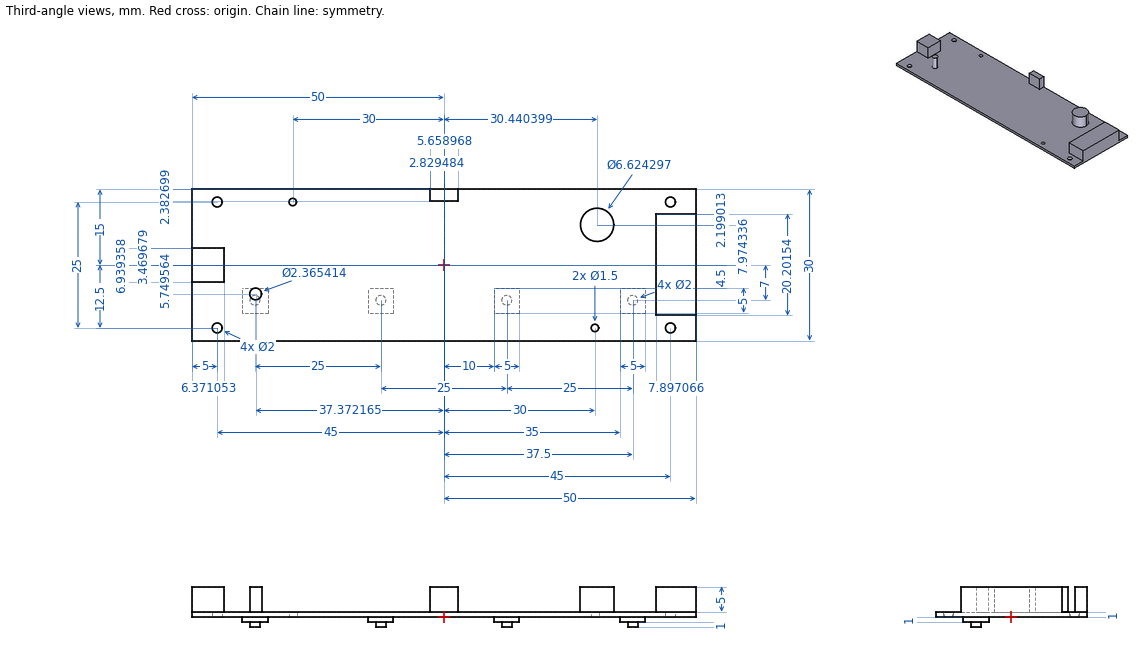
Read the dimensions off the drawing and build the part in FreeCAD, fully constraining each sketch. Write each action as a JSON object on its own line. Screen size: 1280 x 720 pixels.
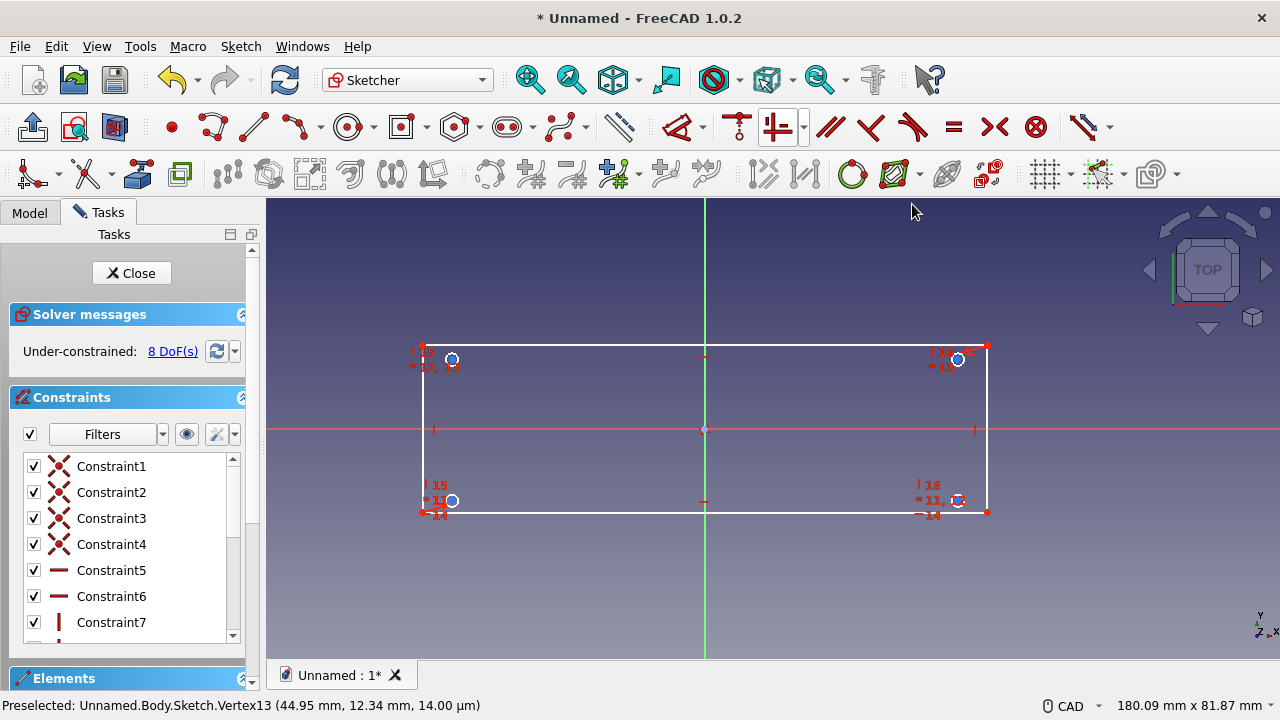
{"action": "scroll", "coordinate": [452, 360], "scroll_direction": "up", "scroll_amount": 4}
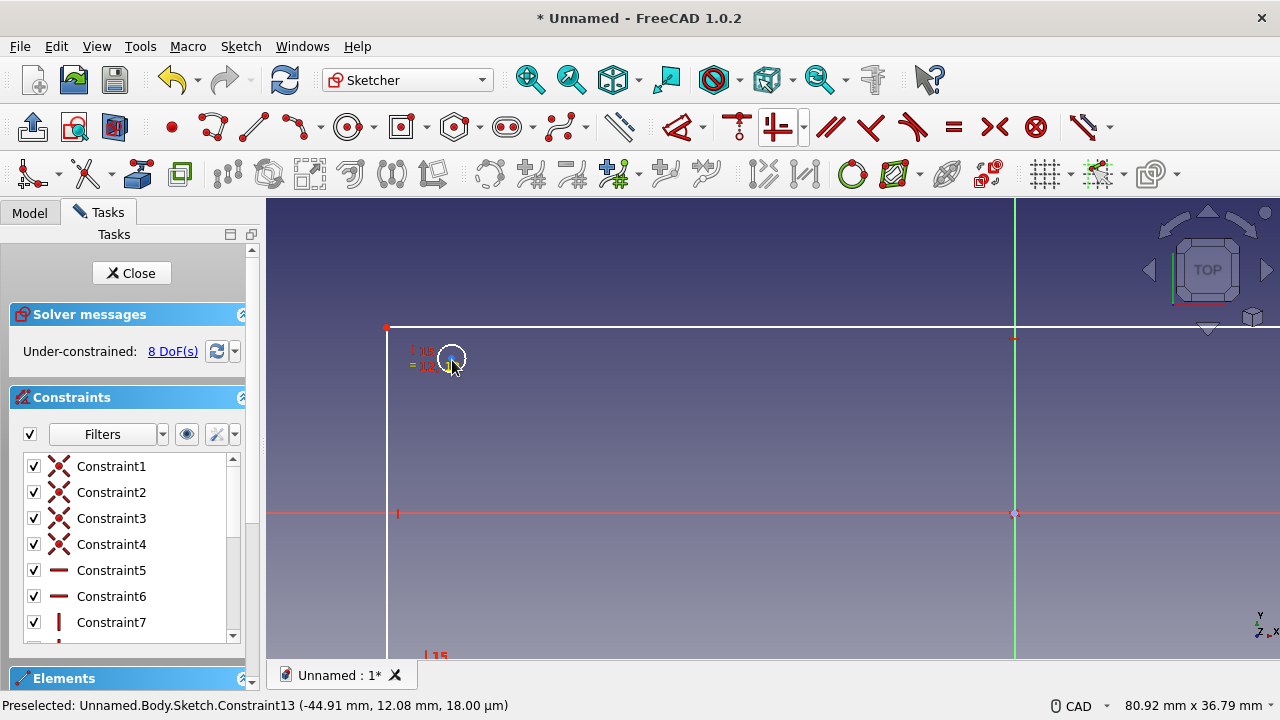
{"action": "scroll", "coordinate": [452, 359], "scroll_direction": "up", "scroll_amount": 4}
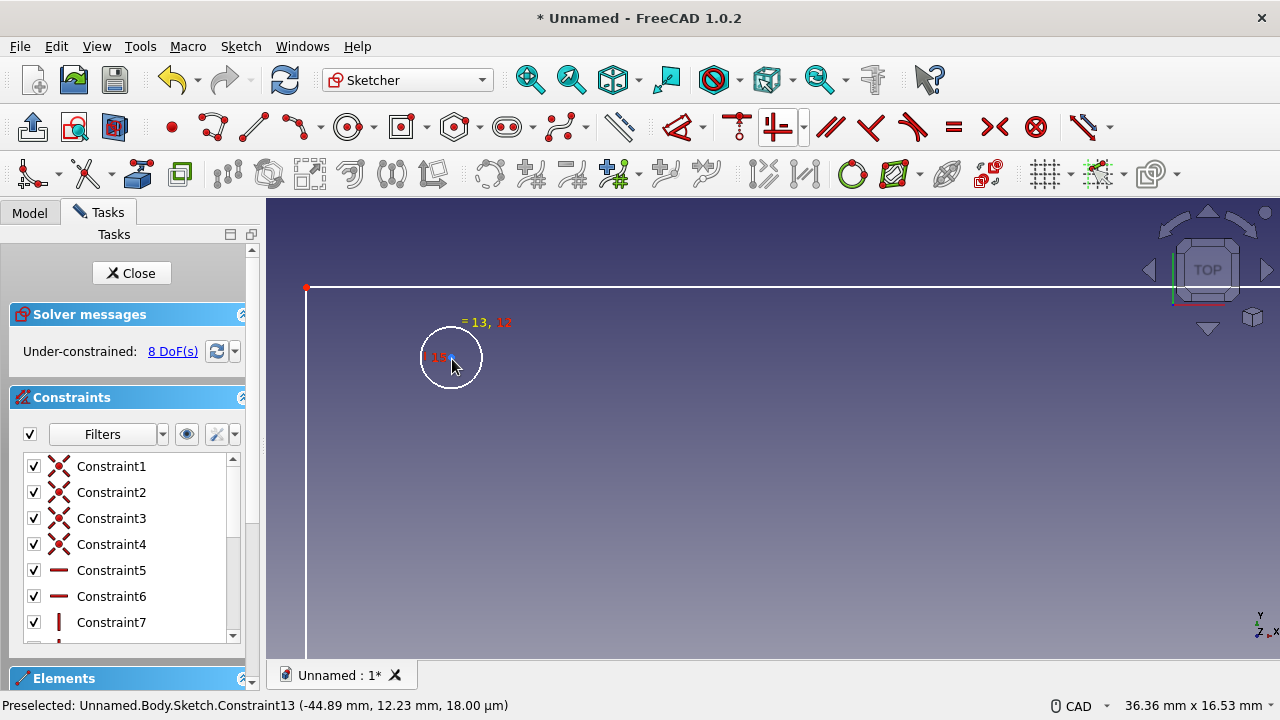
{"action": "left_click", "coordinate": [451, 358]}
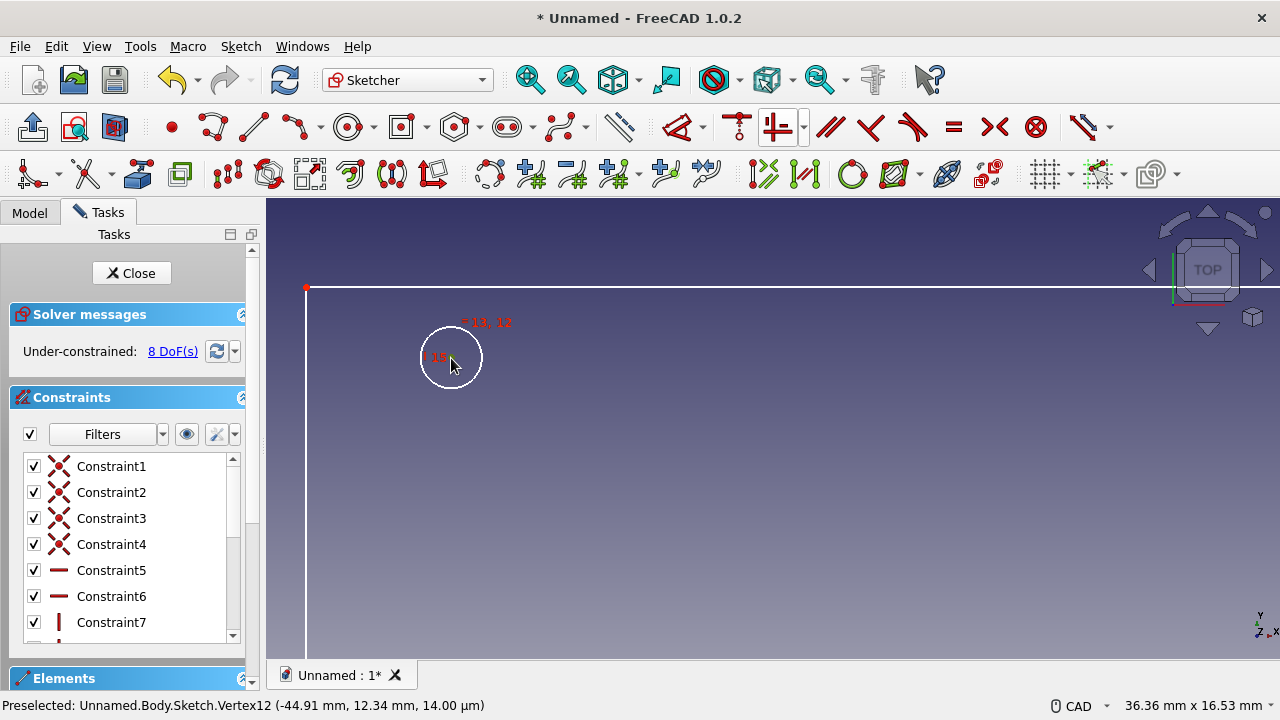
{"action": "scroll", "coordinate": [452, 359], "scroll_direction": "down", "scroll_amount": 8}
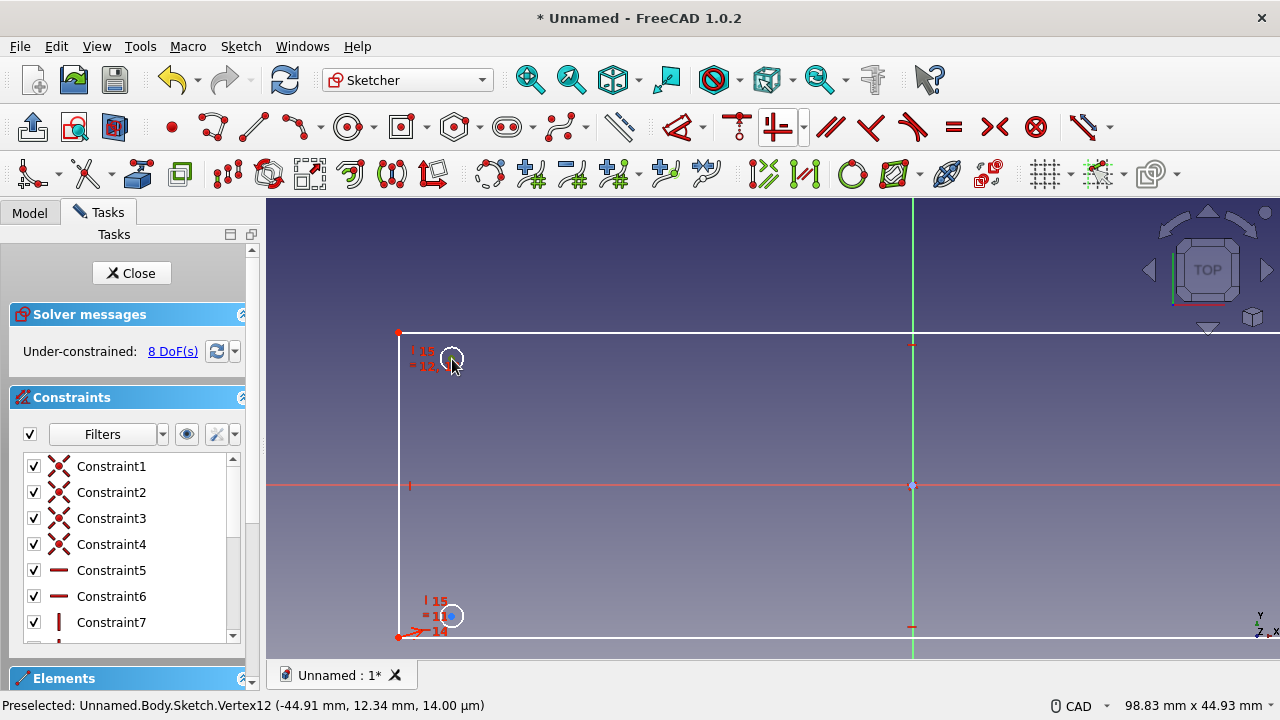
{"action": "left_click", "coordinate": [958, 359]}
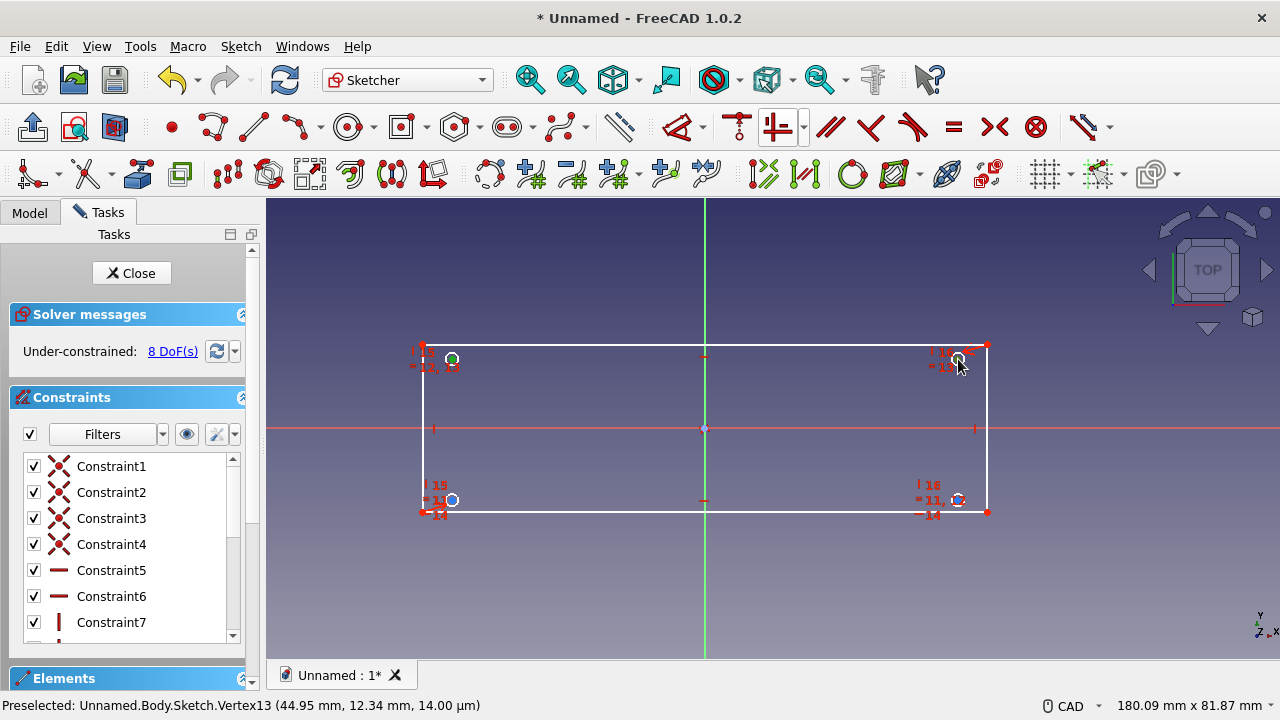
{"action": "key", "text": "h"}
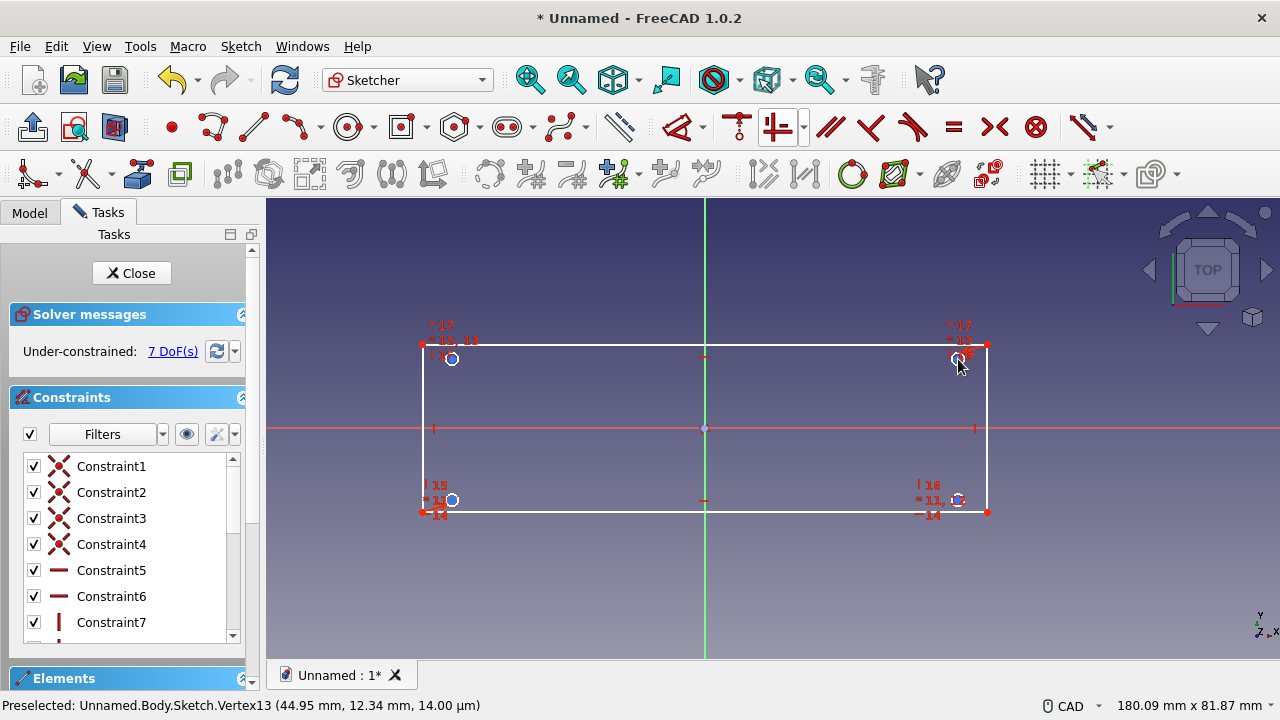
{"action": "left_click", "coordinate": [676, 128]}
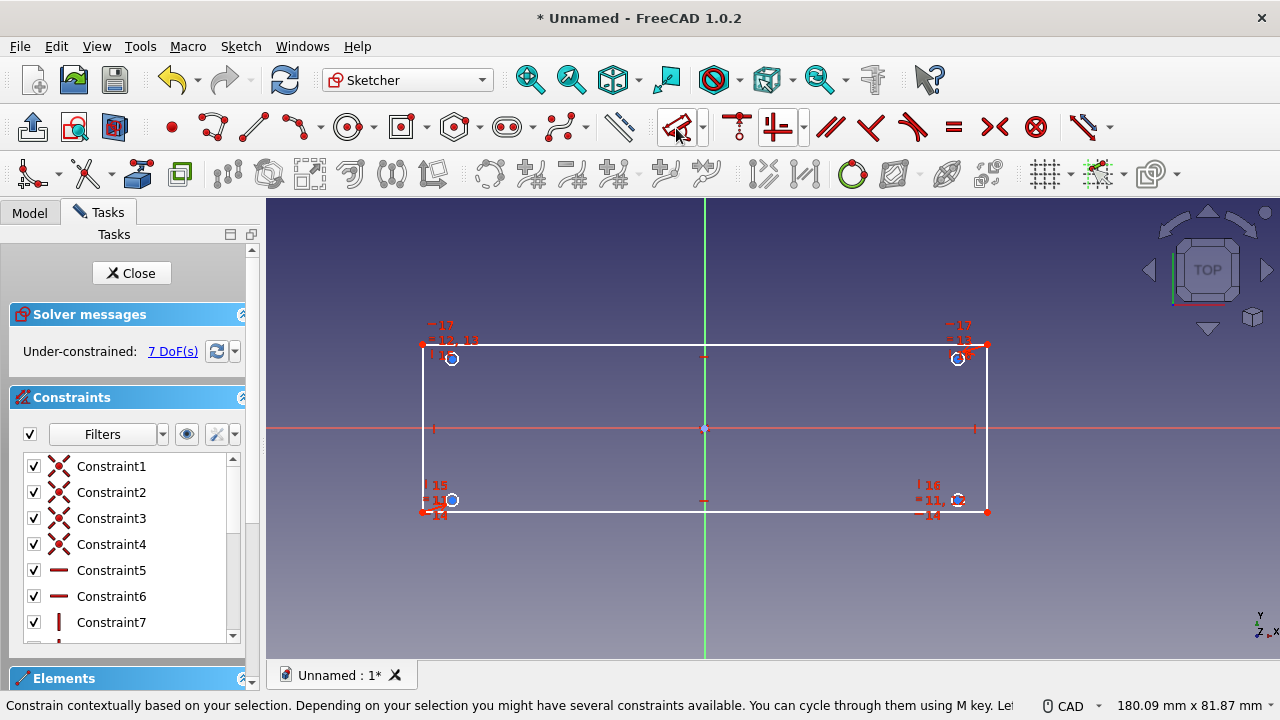
{"action": "scroll", "coordinate": [448, 496], "scroll_direction": "up", "scroll_amount": 7}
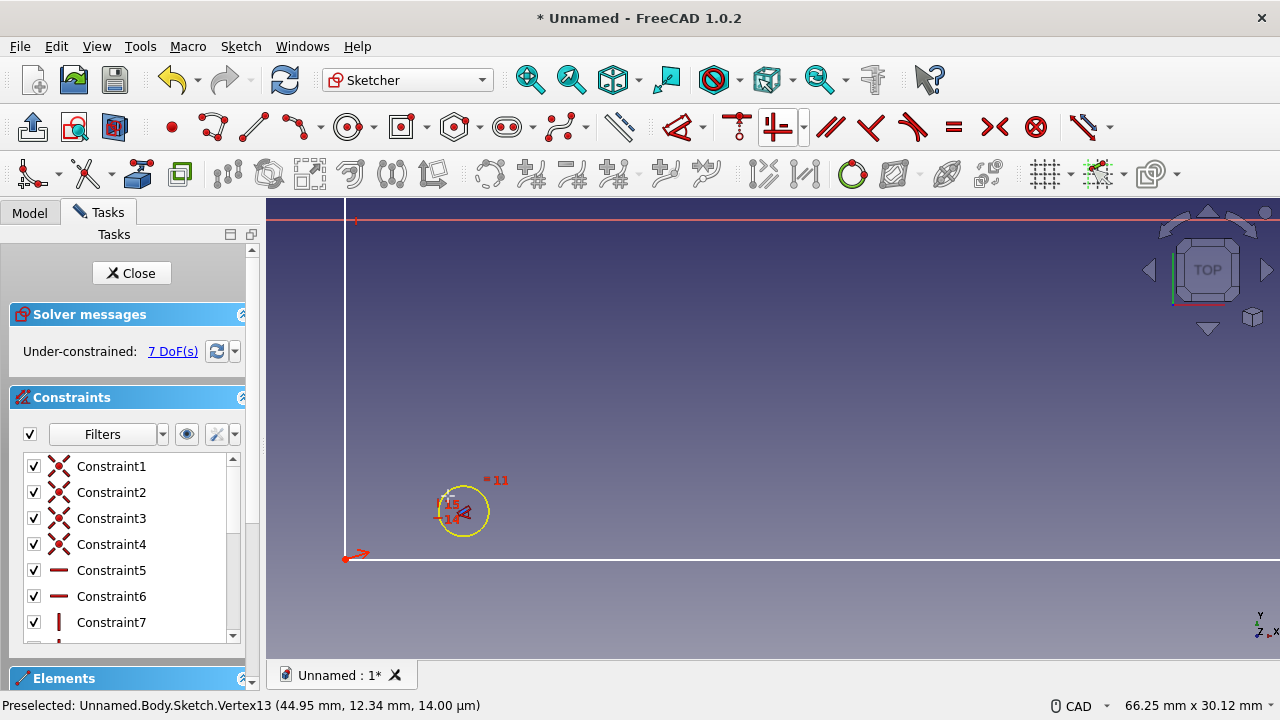
{"action": "left_click", "coordinate": [446, 494]}
{"action": "left_click", "coordinate": [423, 472]}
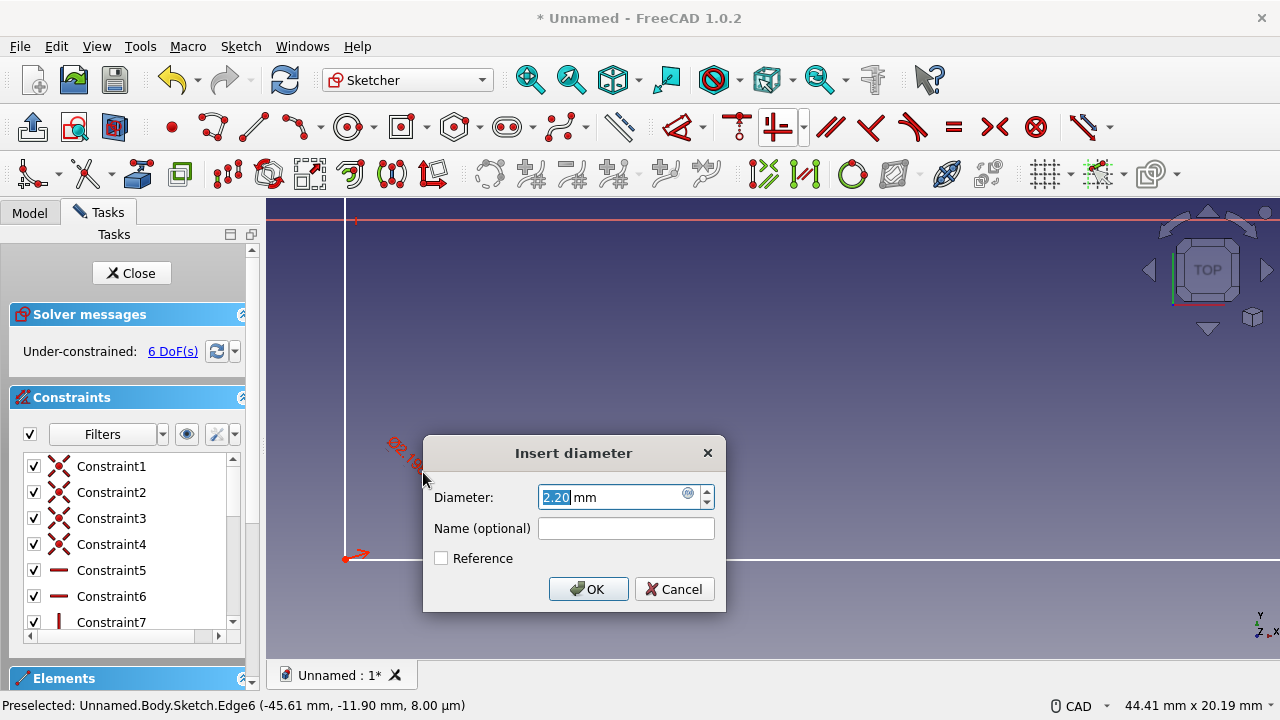
{"action": "type", "text": "2"}
{"action": "key", "text": "Return"}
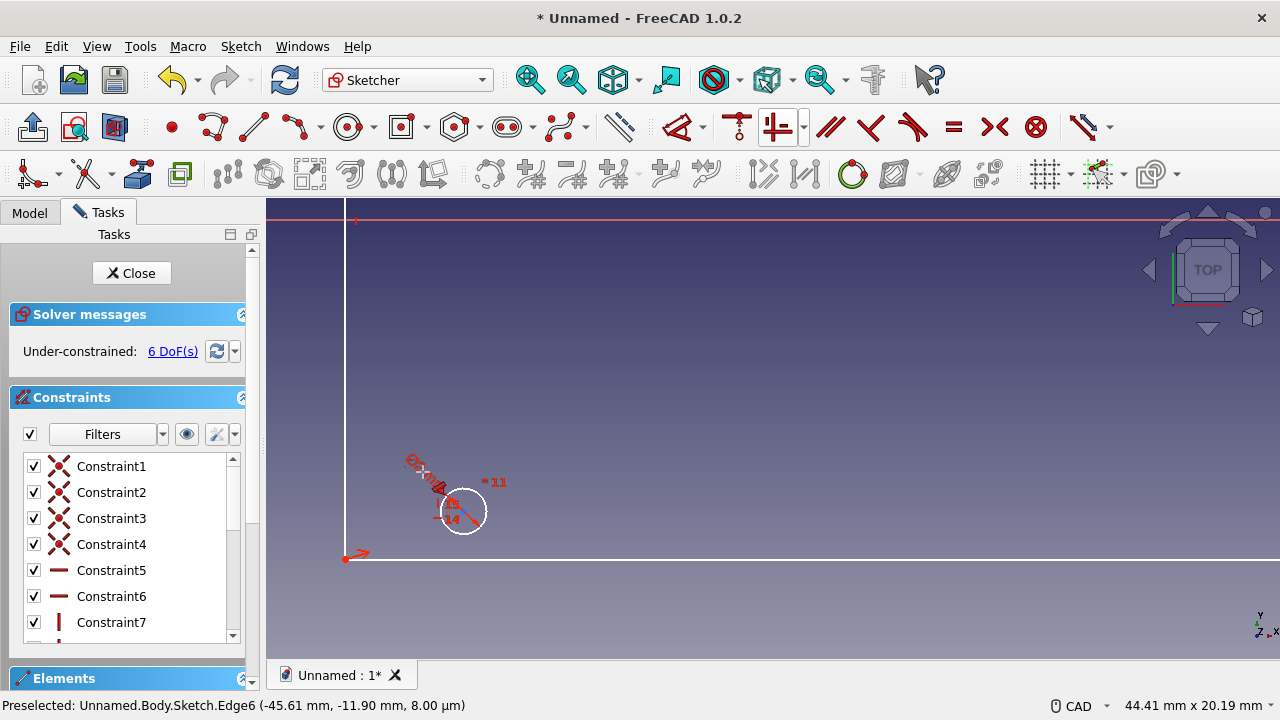
{"action": "scroll", "coordinate": [448, 497], "scroll_direction": "down", "scroll_amount": 7}